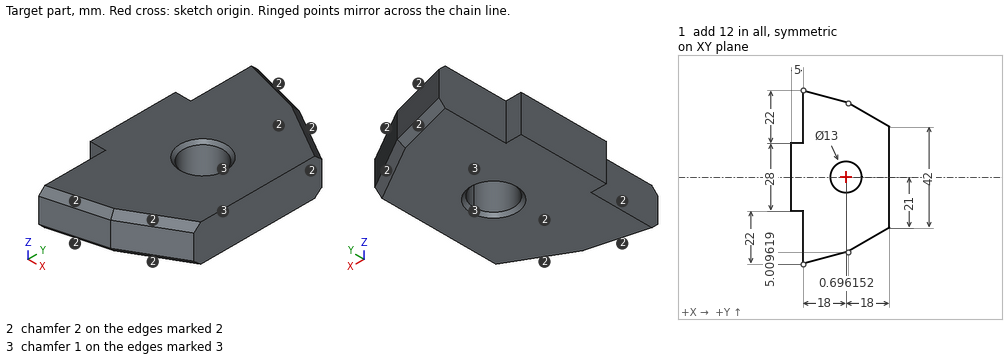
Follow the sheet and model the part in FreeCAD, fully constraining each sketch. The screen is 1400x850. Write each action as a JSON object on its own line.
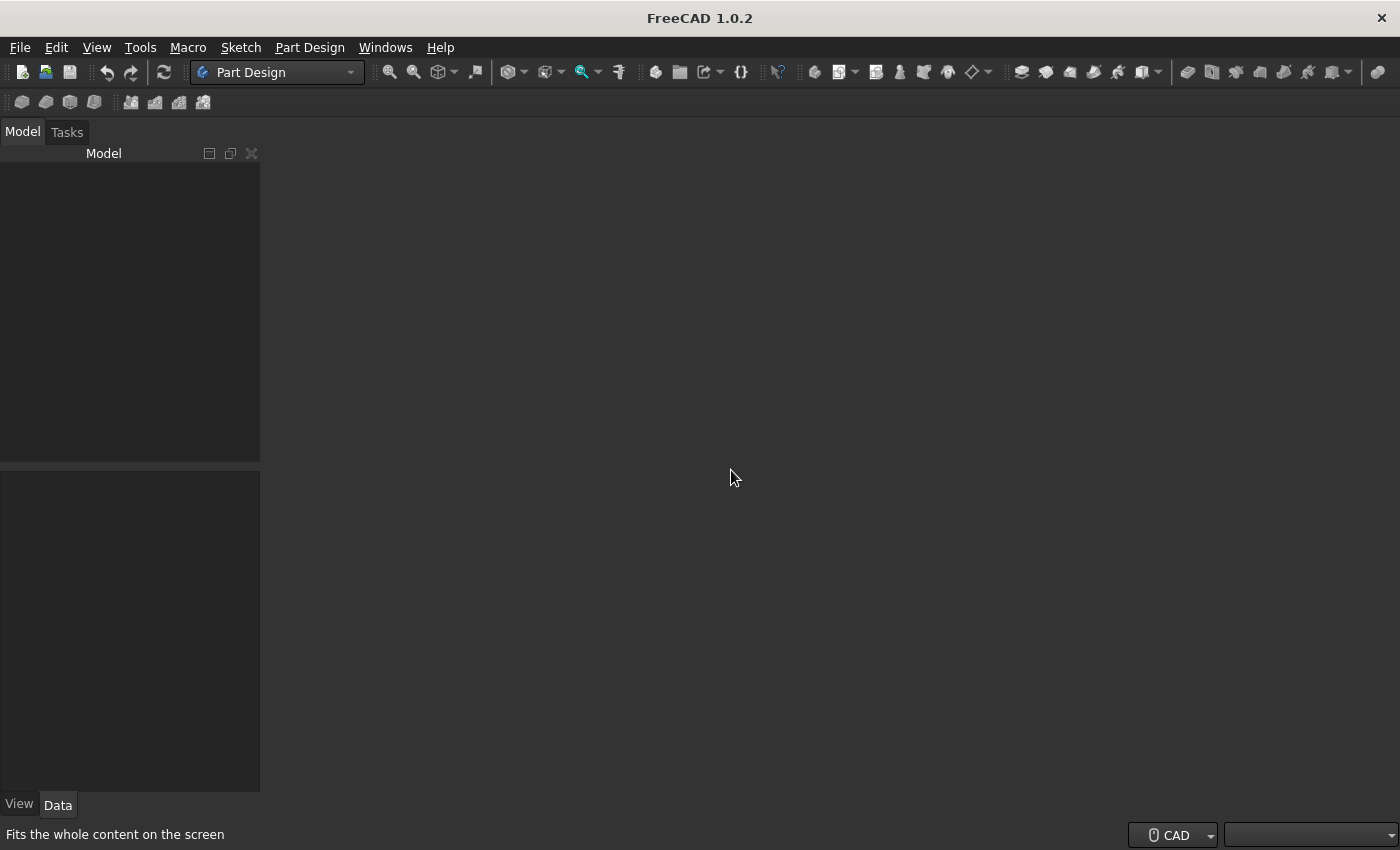
{"action": "left_click", "coordinate": [22, 72]}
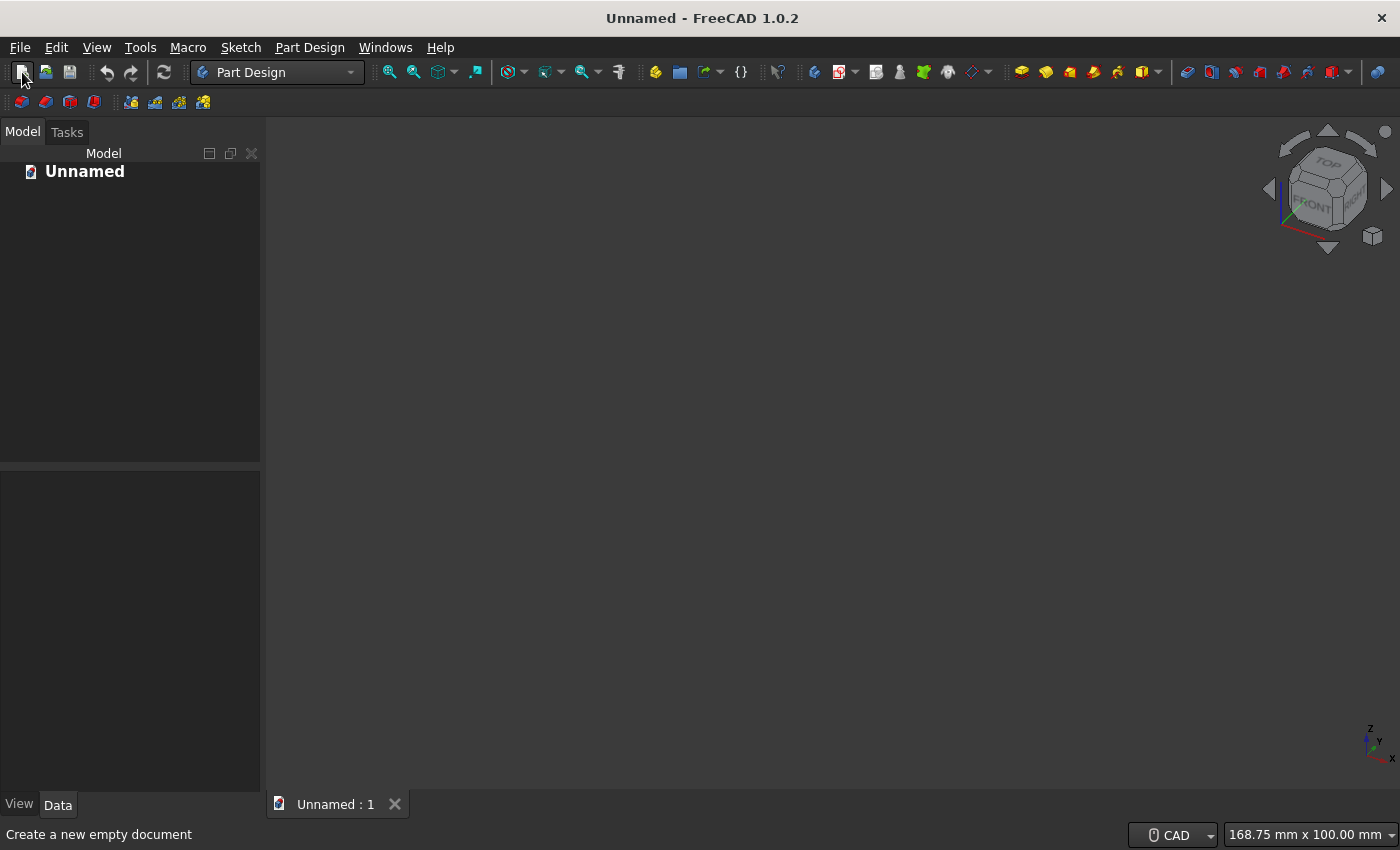
{"action": "left_click", "coordinate": [840, 72]}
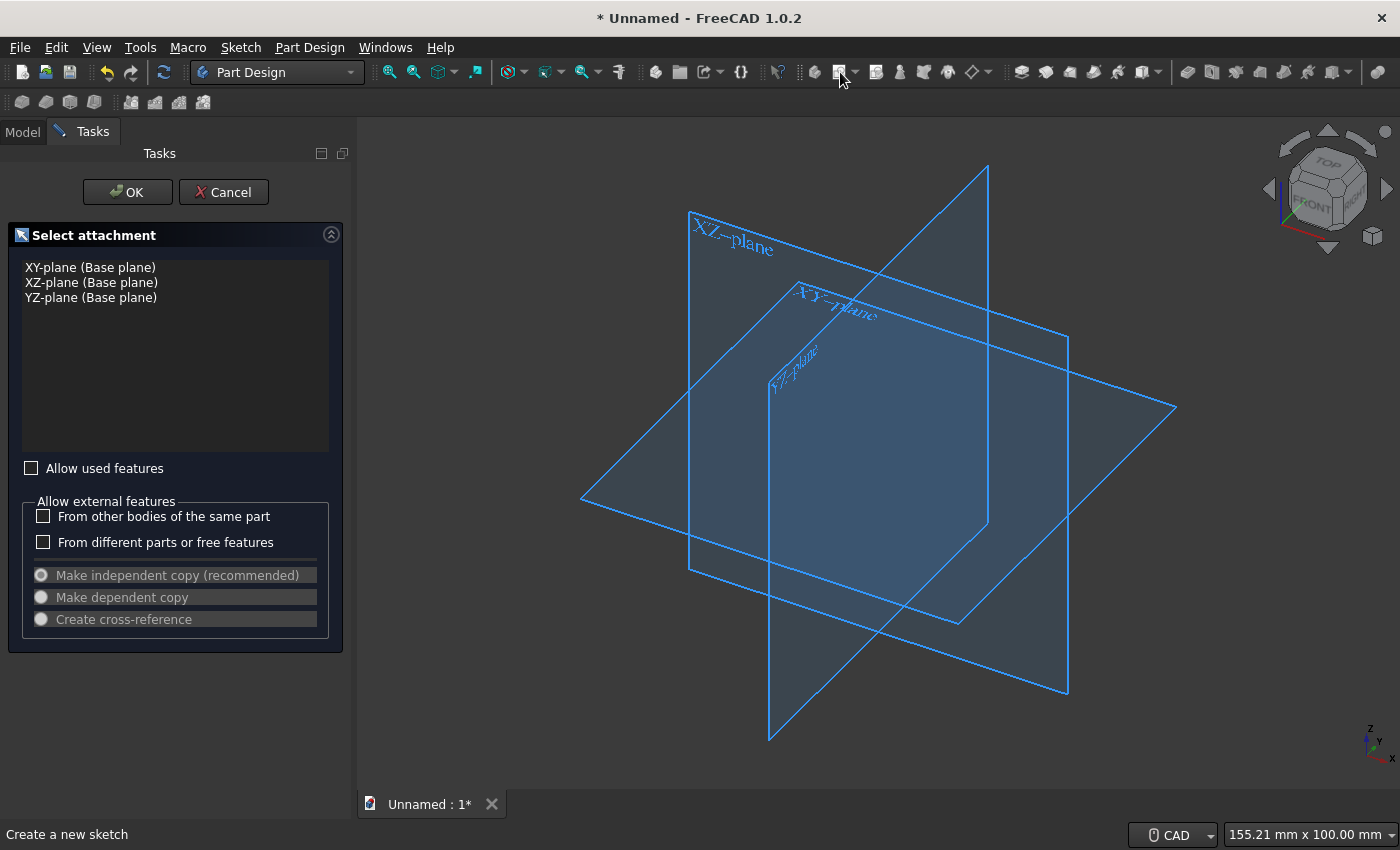
{"action": "left_click", "coordinate": [82, 268]}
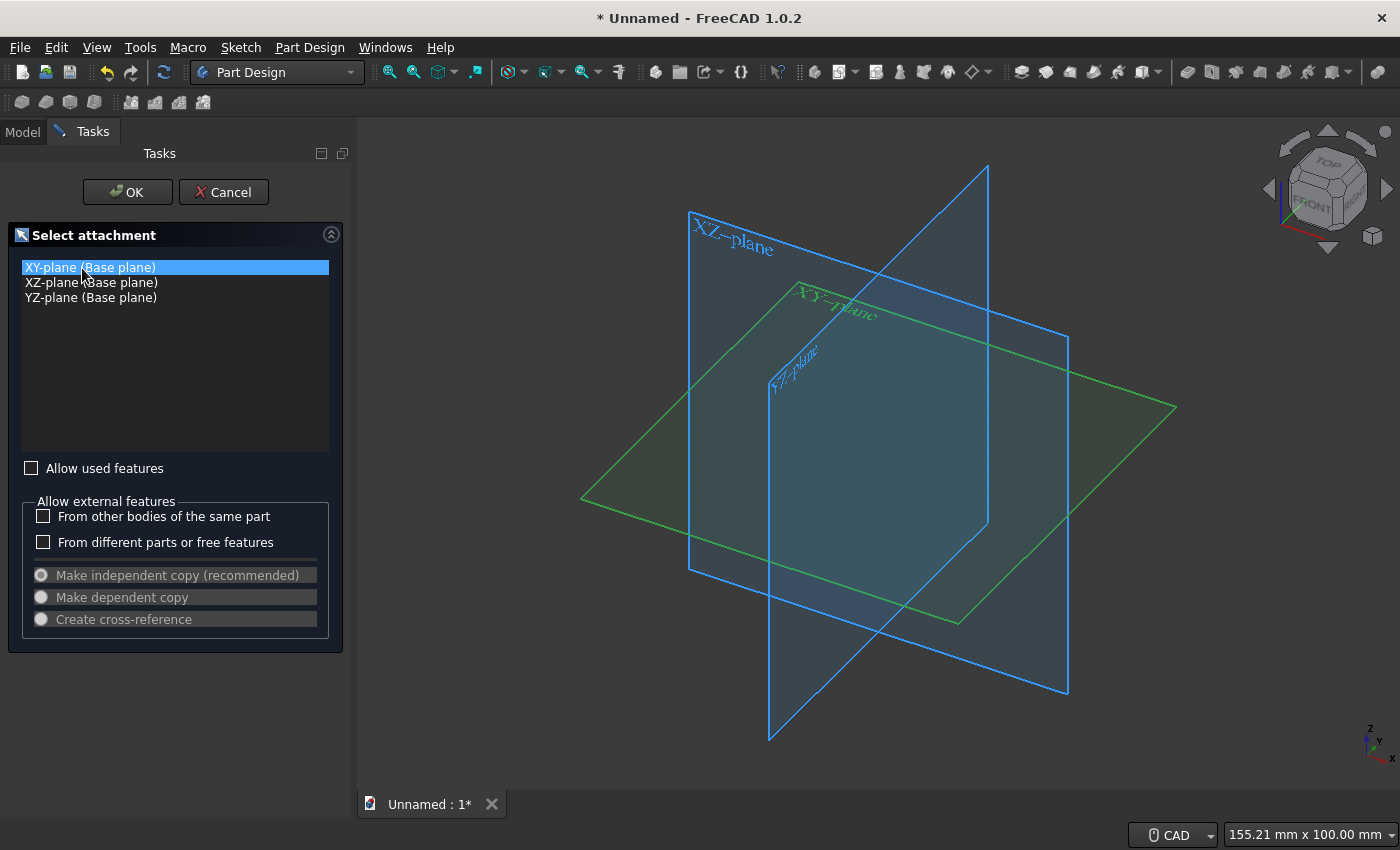
{"action": "left_click", "coordinate": [128, 192]}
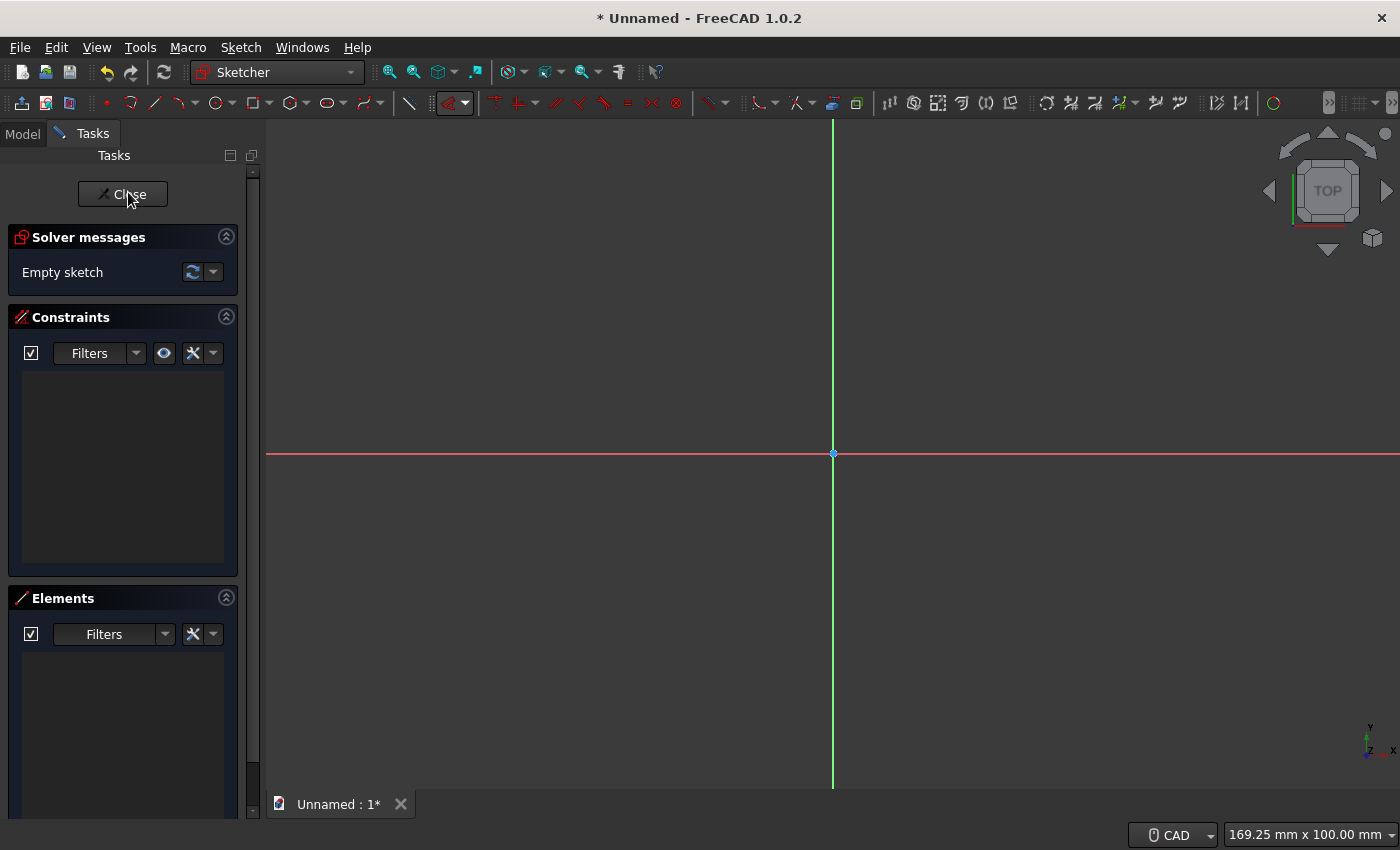
{"action": "left_click", "coordinate": [132, 104]}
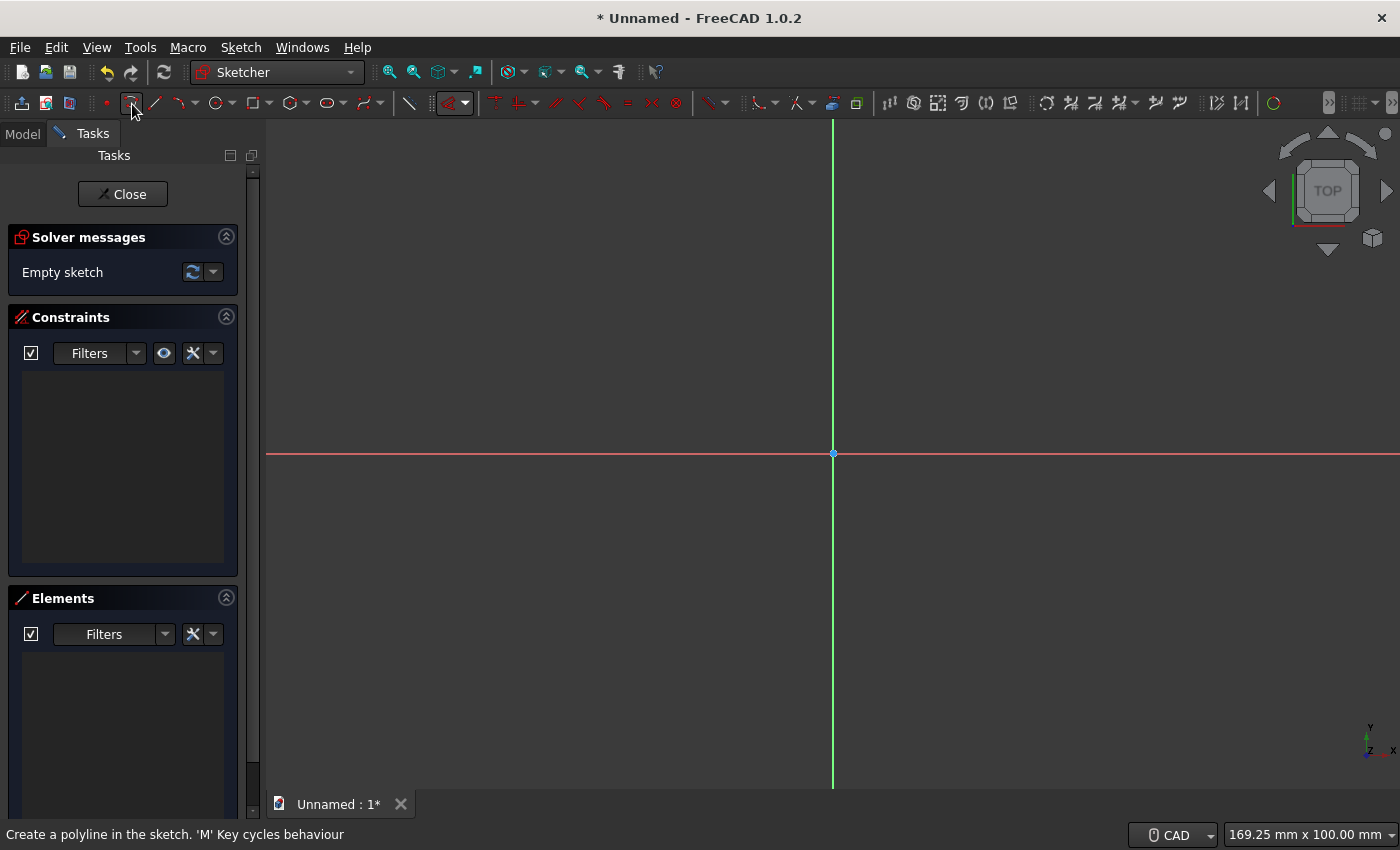
{"action": "left_click", "coordinate": [712, 548]}
{"action": "left_click", "coordinate": [712, 695]}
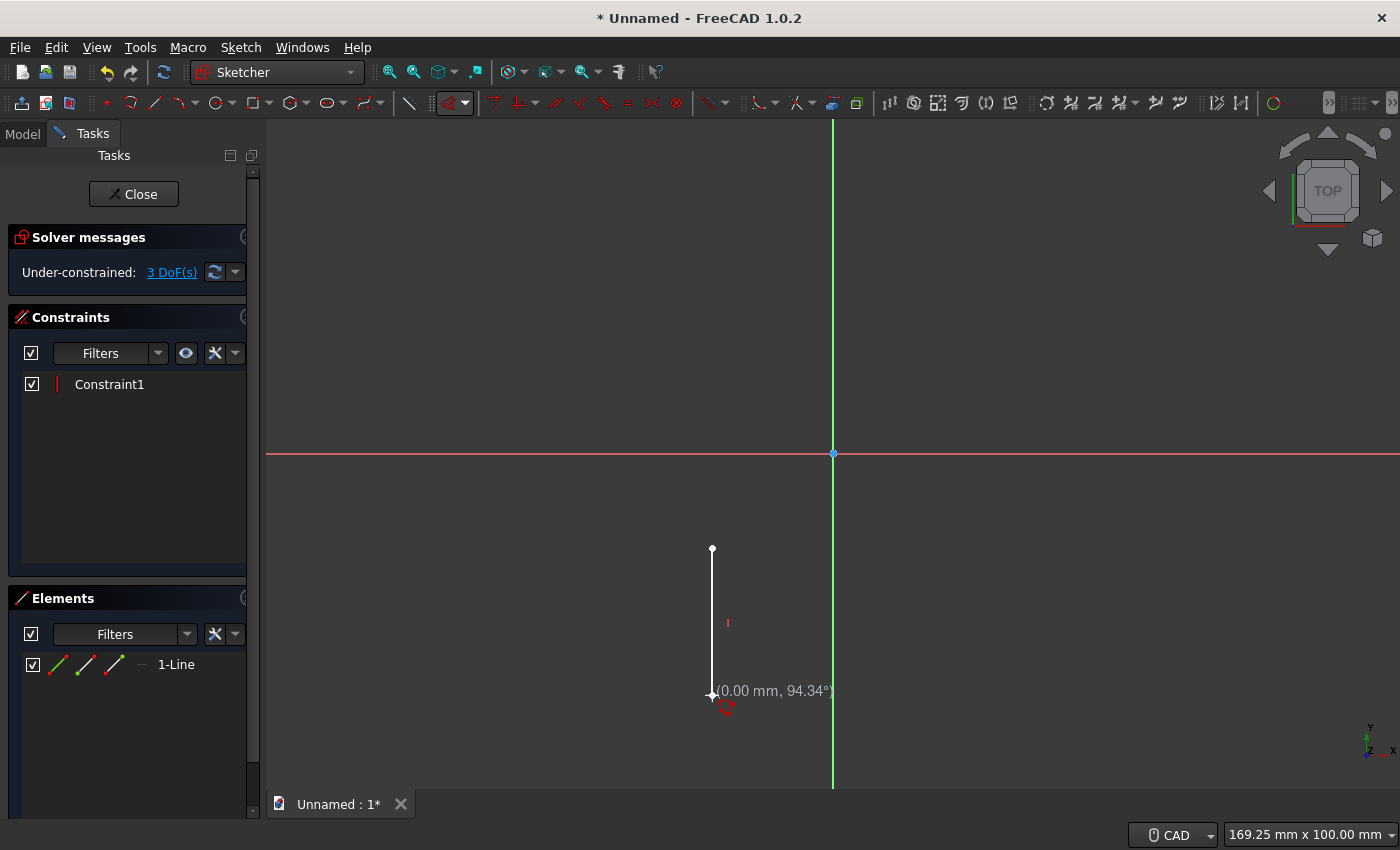
{"action": "scroll", "coordinate": [838, 662], "scroll_direction": "up", "scroll_amount": 7}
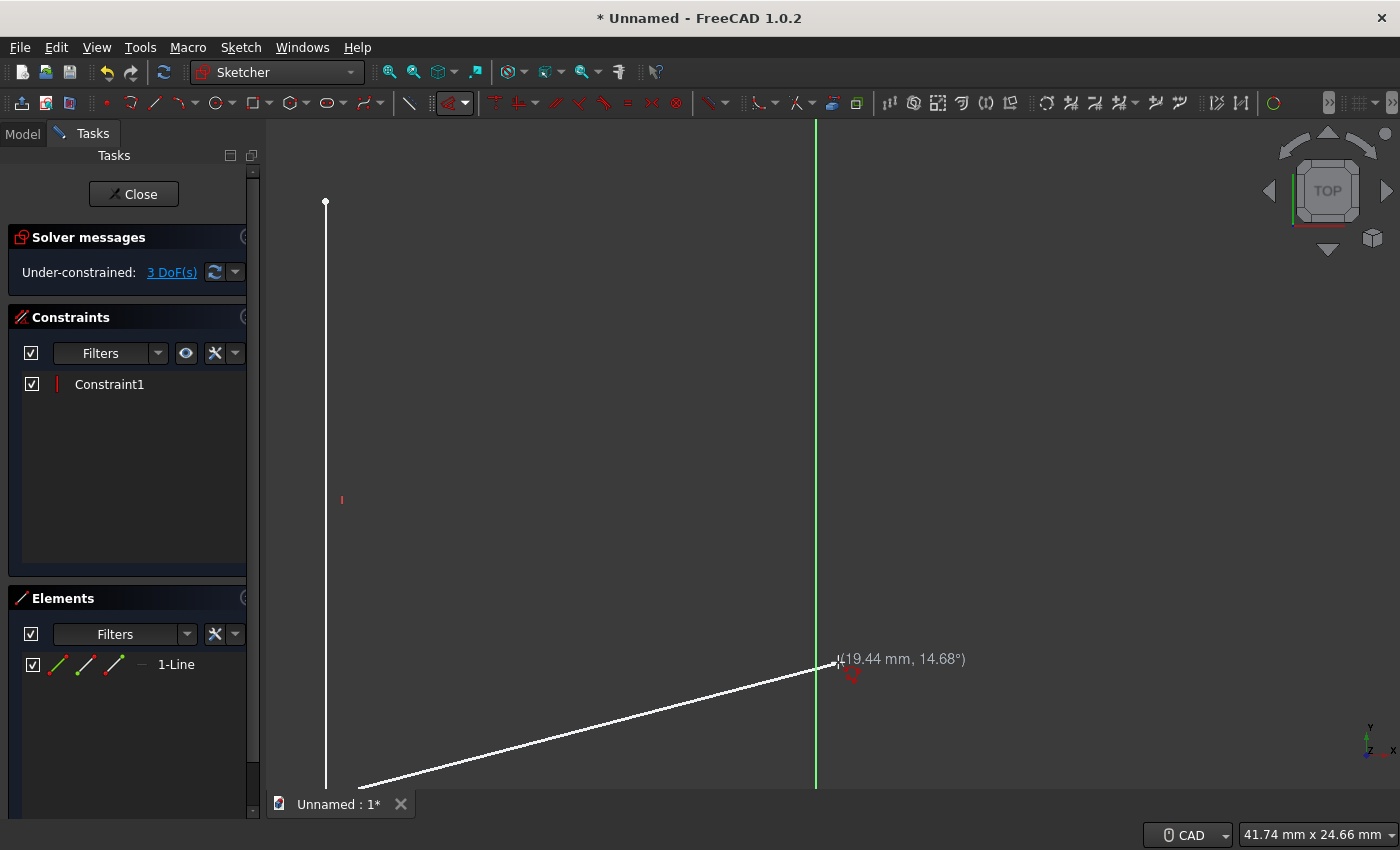
{"action": "left_click", "coordinate": [835, 658]}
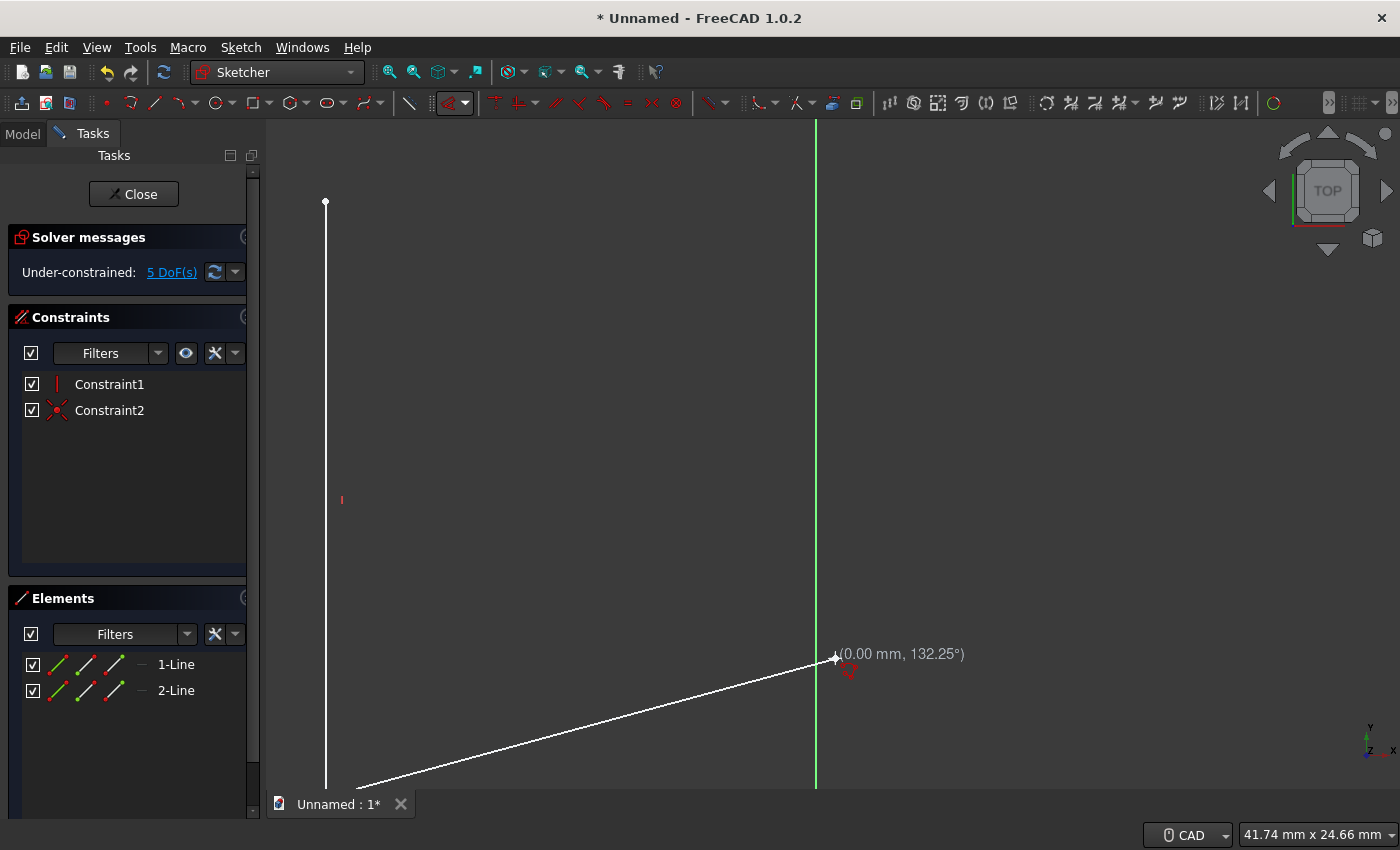
{"action": "scroll", "coordinate": [769, 615], "scroll_direction": "down", "scroll_amount": 8}